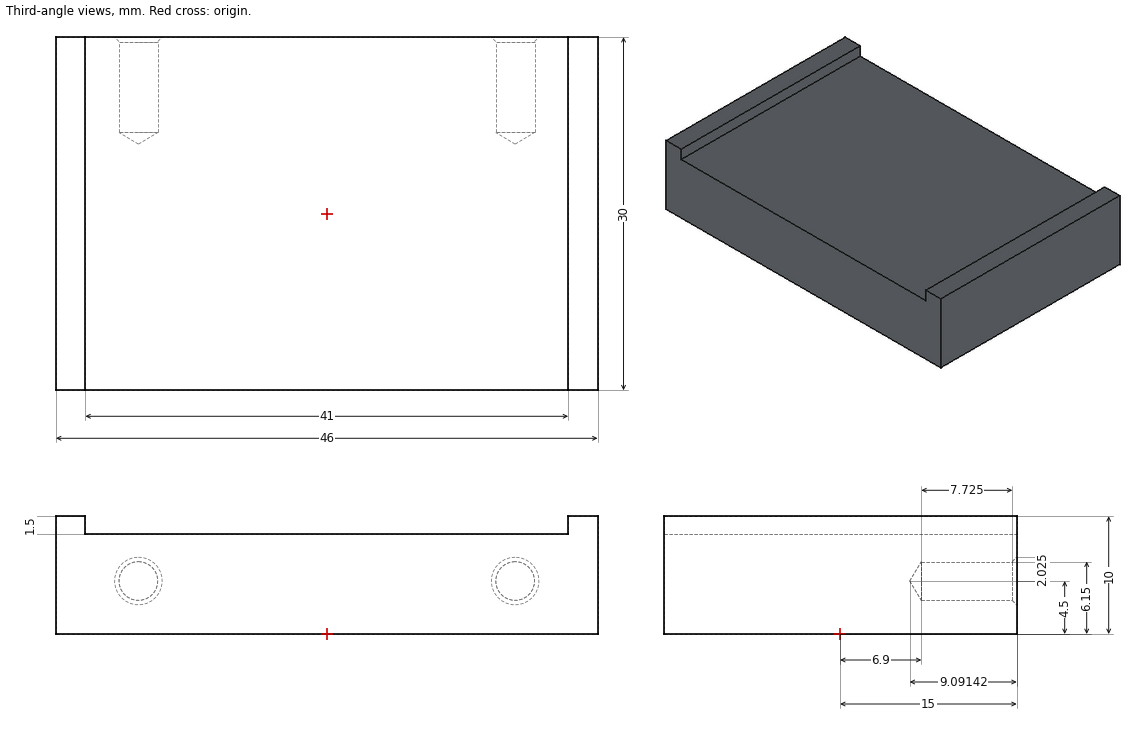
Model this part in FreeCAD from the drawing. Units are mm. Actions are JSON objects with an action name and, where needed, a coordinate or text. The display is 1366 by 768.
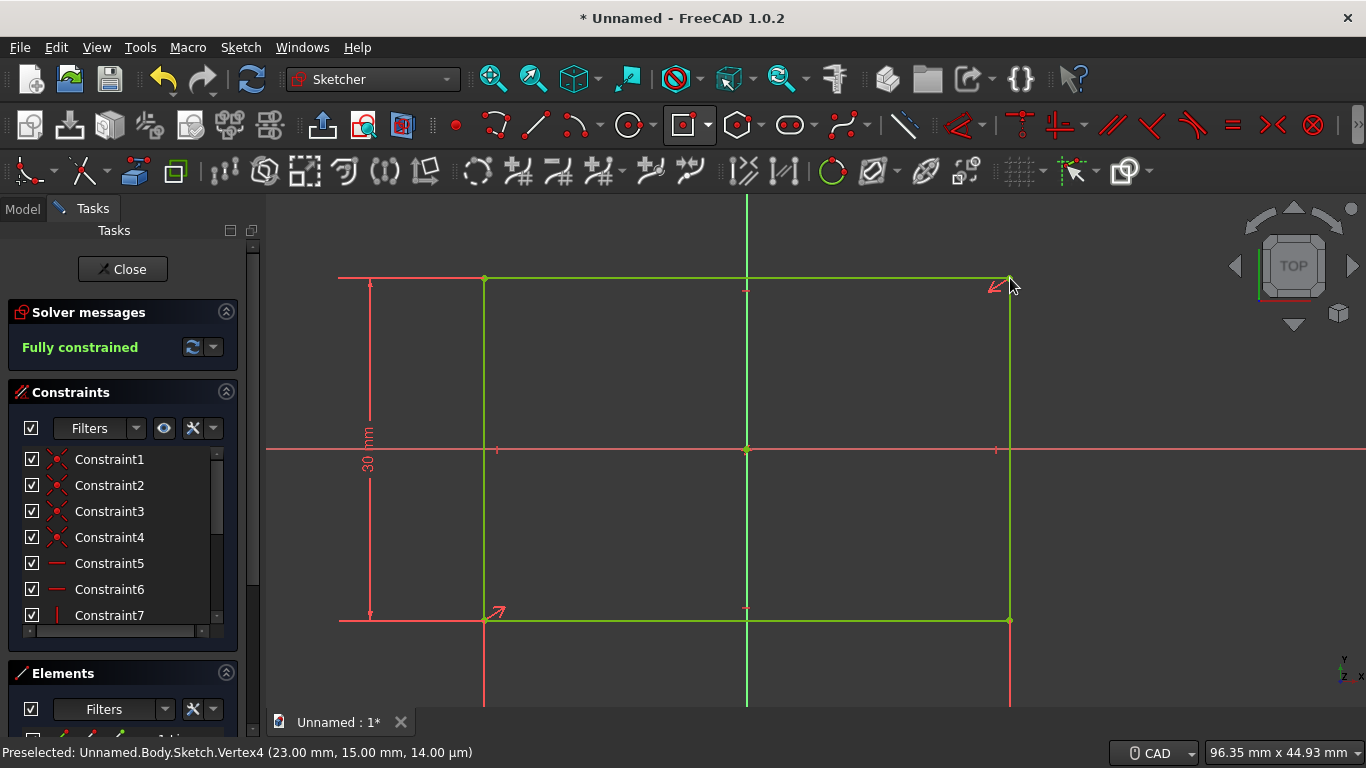
{"action": "left_click", "coordinate": [123, 269]}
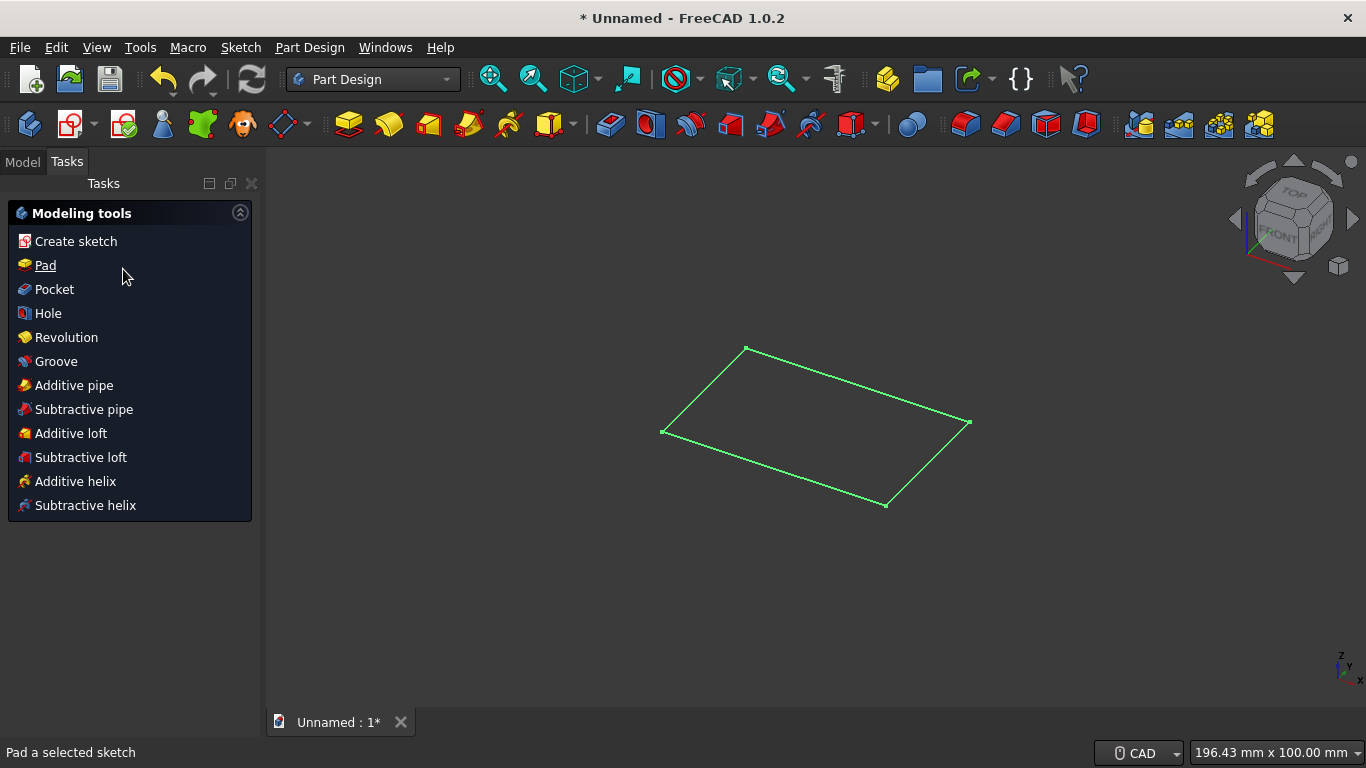
{"action": "left_click", "coordinate": [350, 124]}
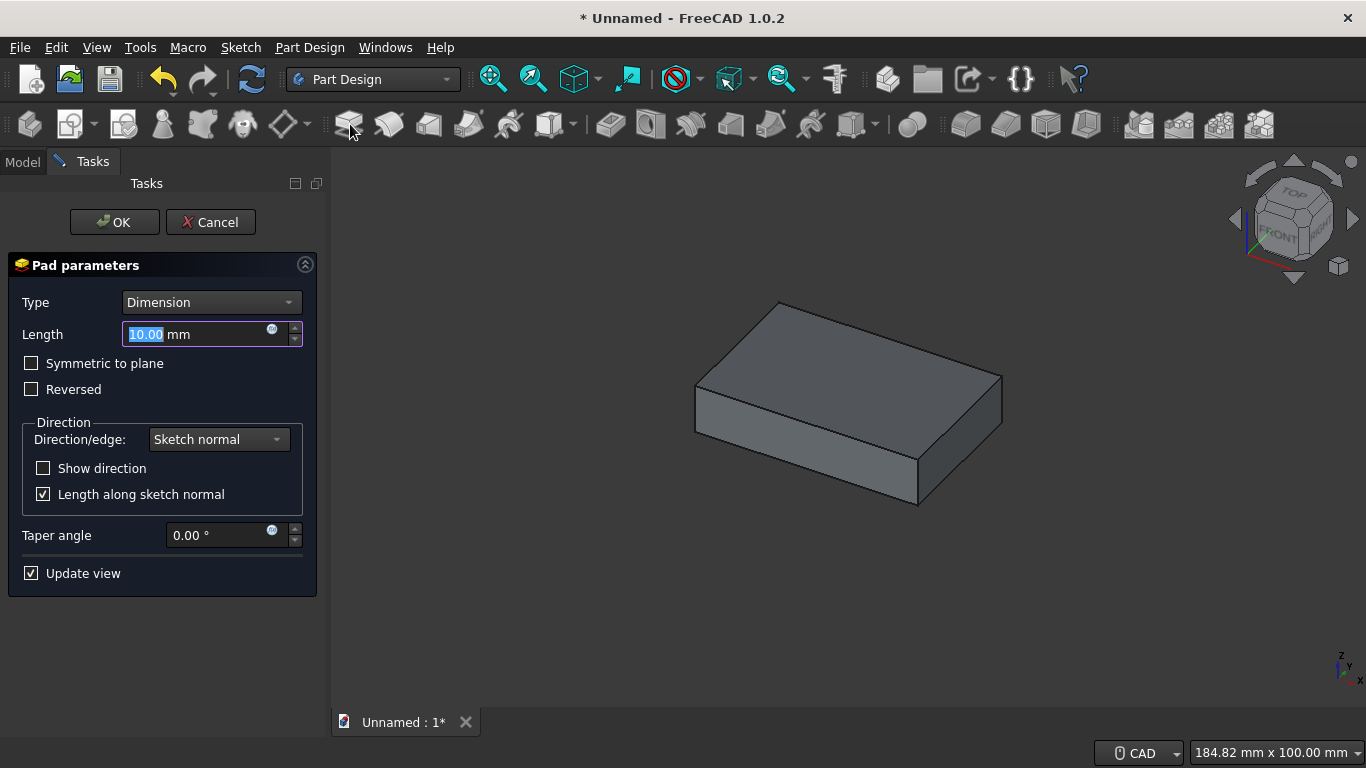
{"action": "type", "text": "10"}
{"action": "key", "text": "Tab"}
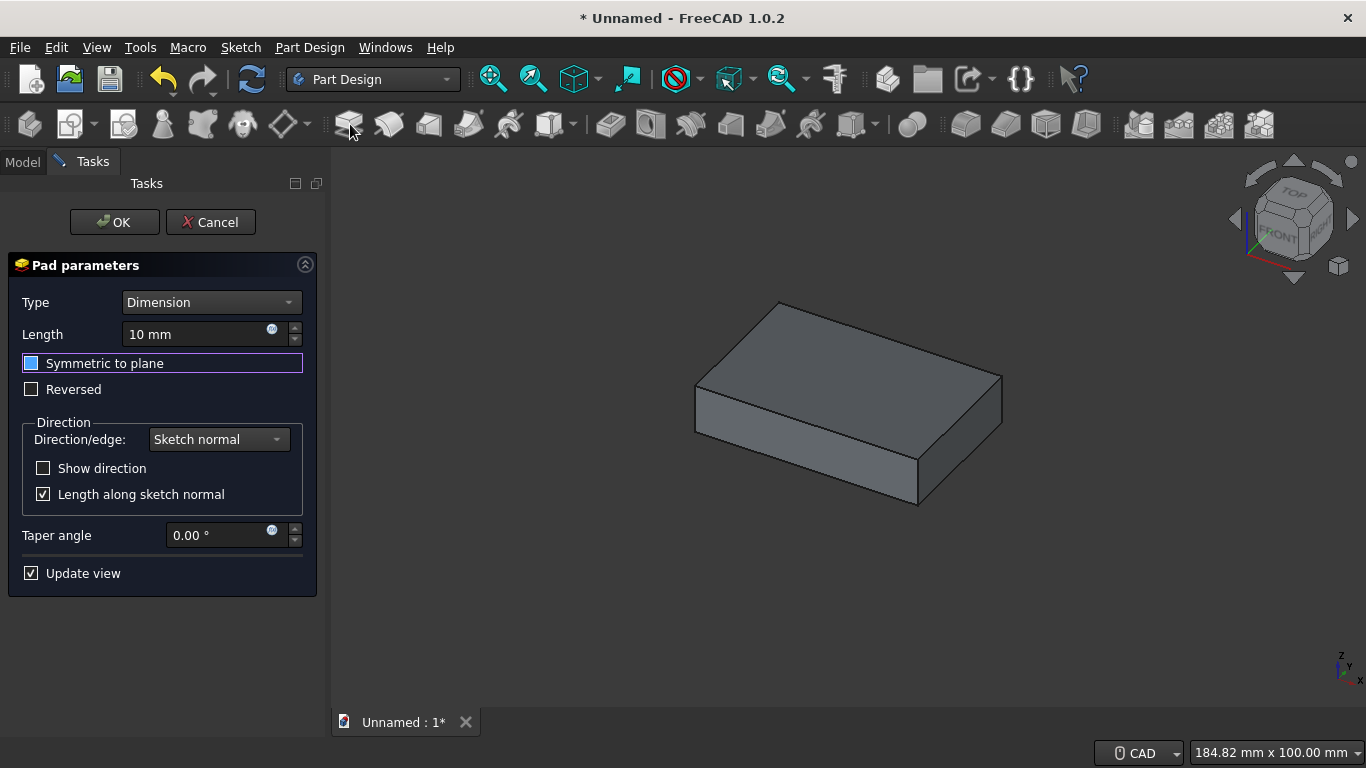
{"action": "left_click", "coordinate": [115, 222]}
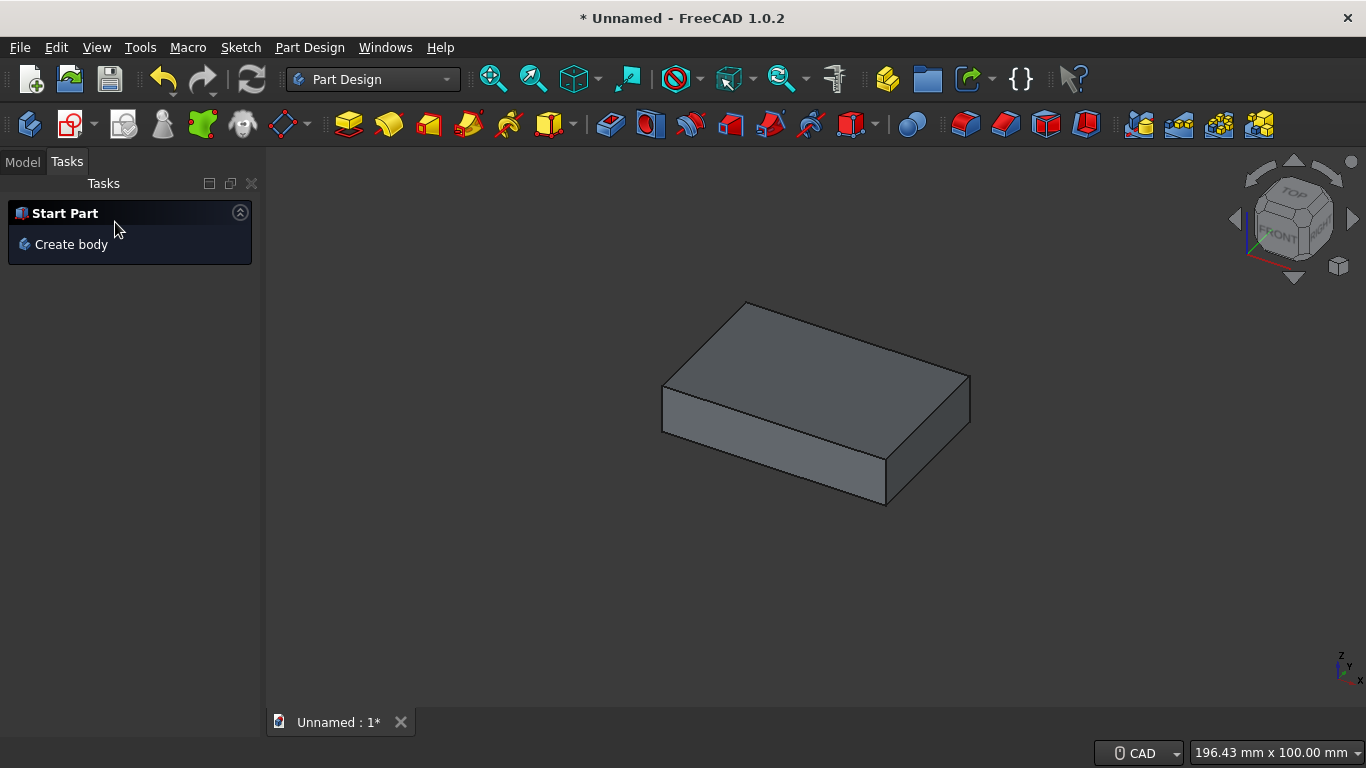
{"action": "key", "text": "v f"}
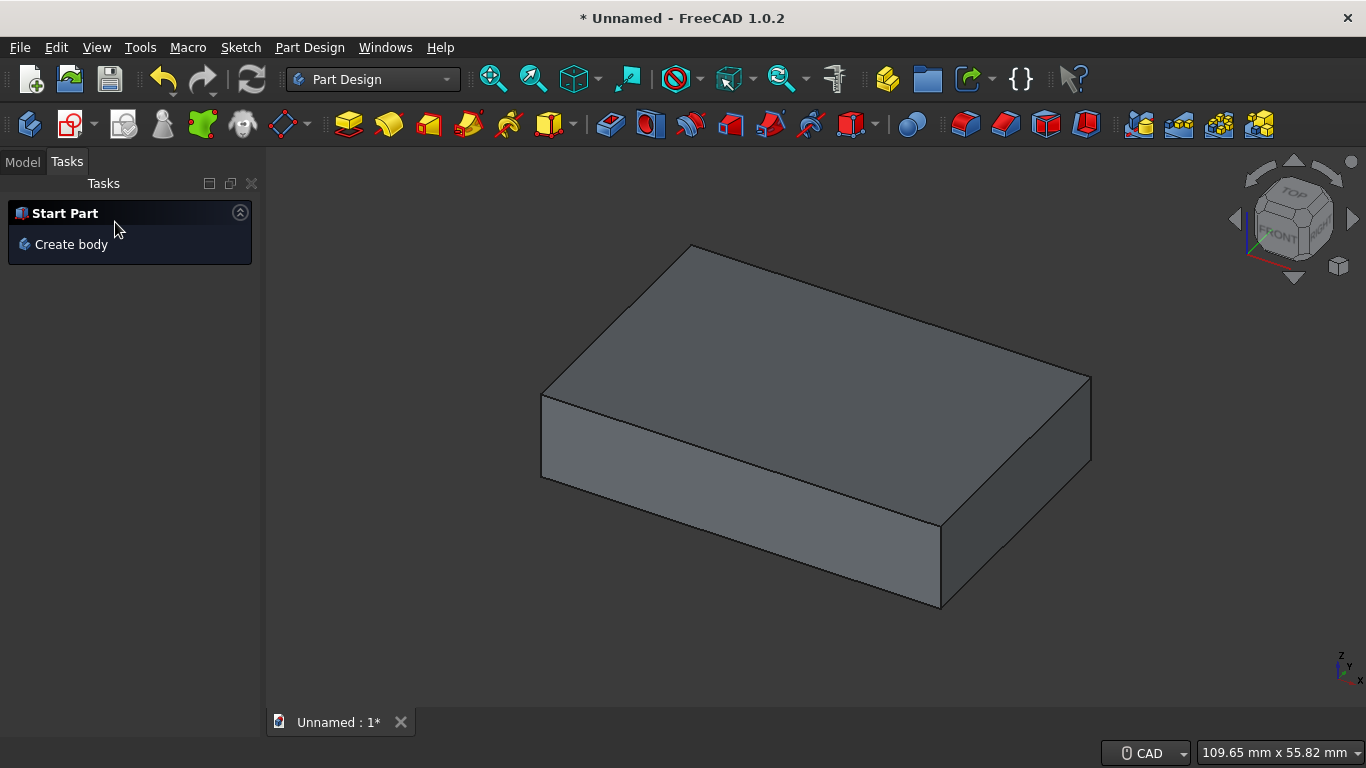
{"action": "left_click", "coordinate": [873, 404]}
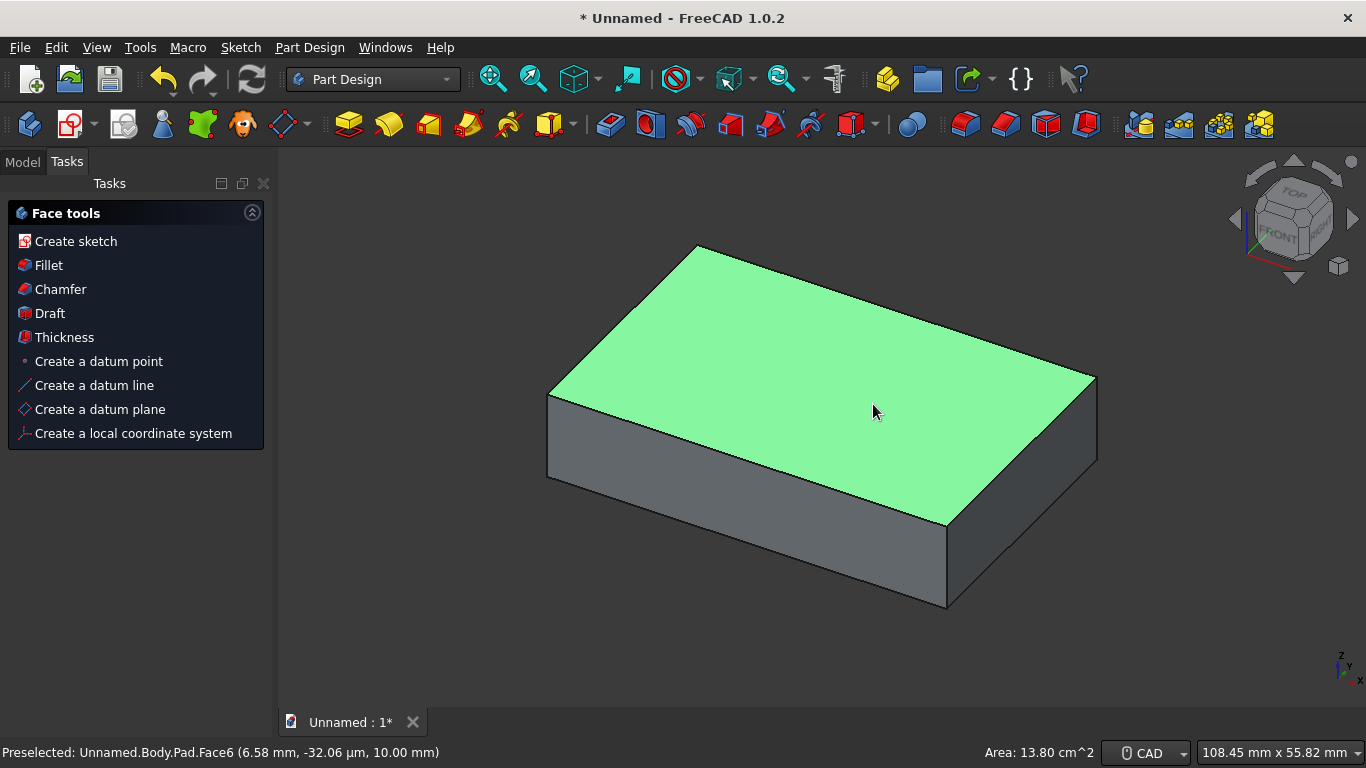
{"action": "left_click", "coordinate": [70, 124]}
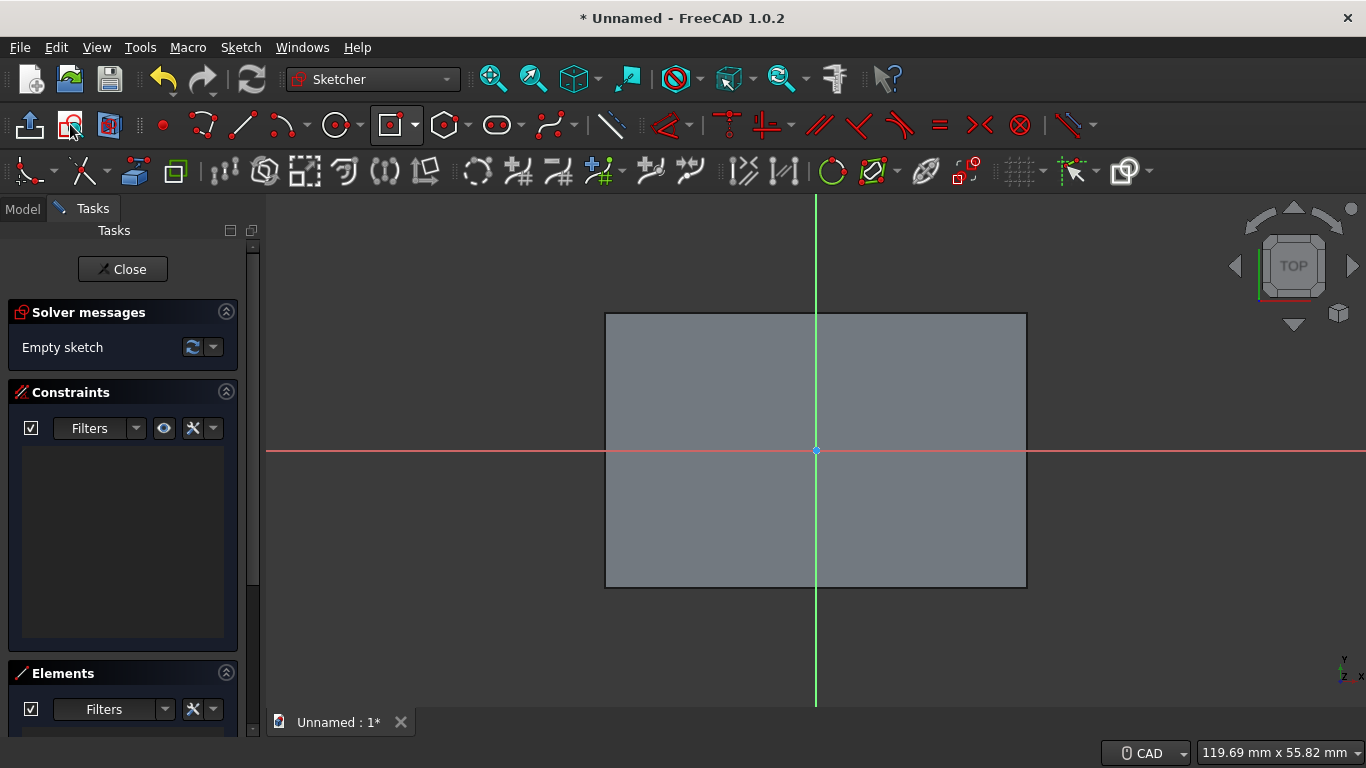
{"action": "left_click", "coordinate": [390, 126]}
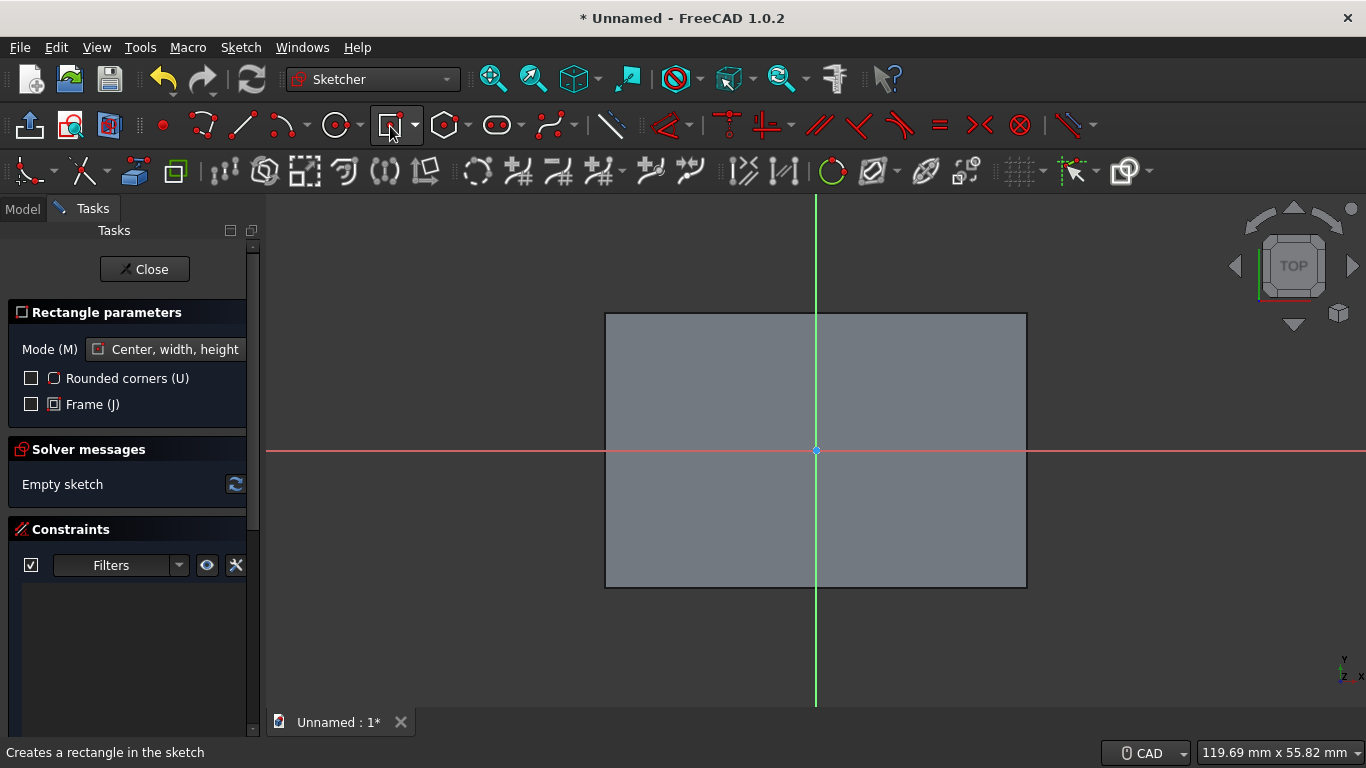
{"action": "left_click", "coordinate": [816, 450]}
{"action": "mouse_move", "coordinate": [1004, 313]}